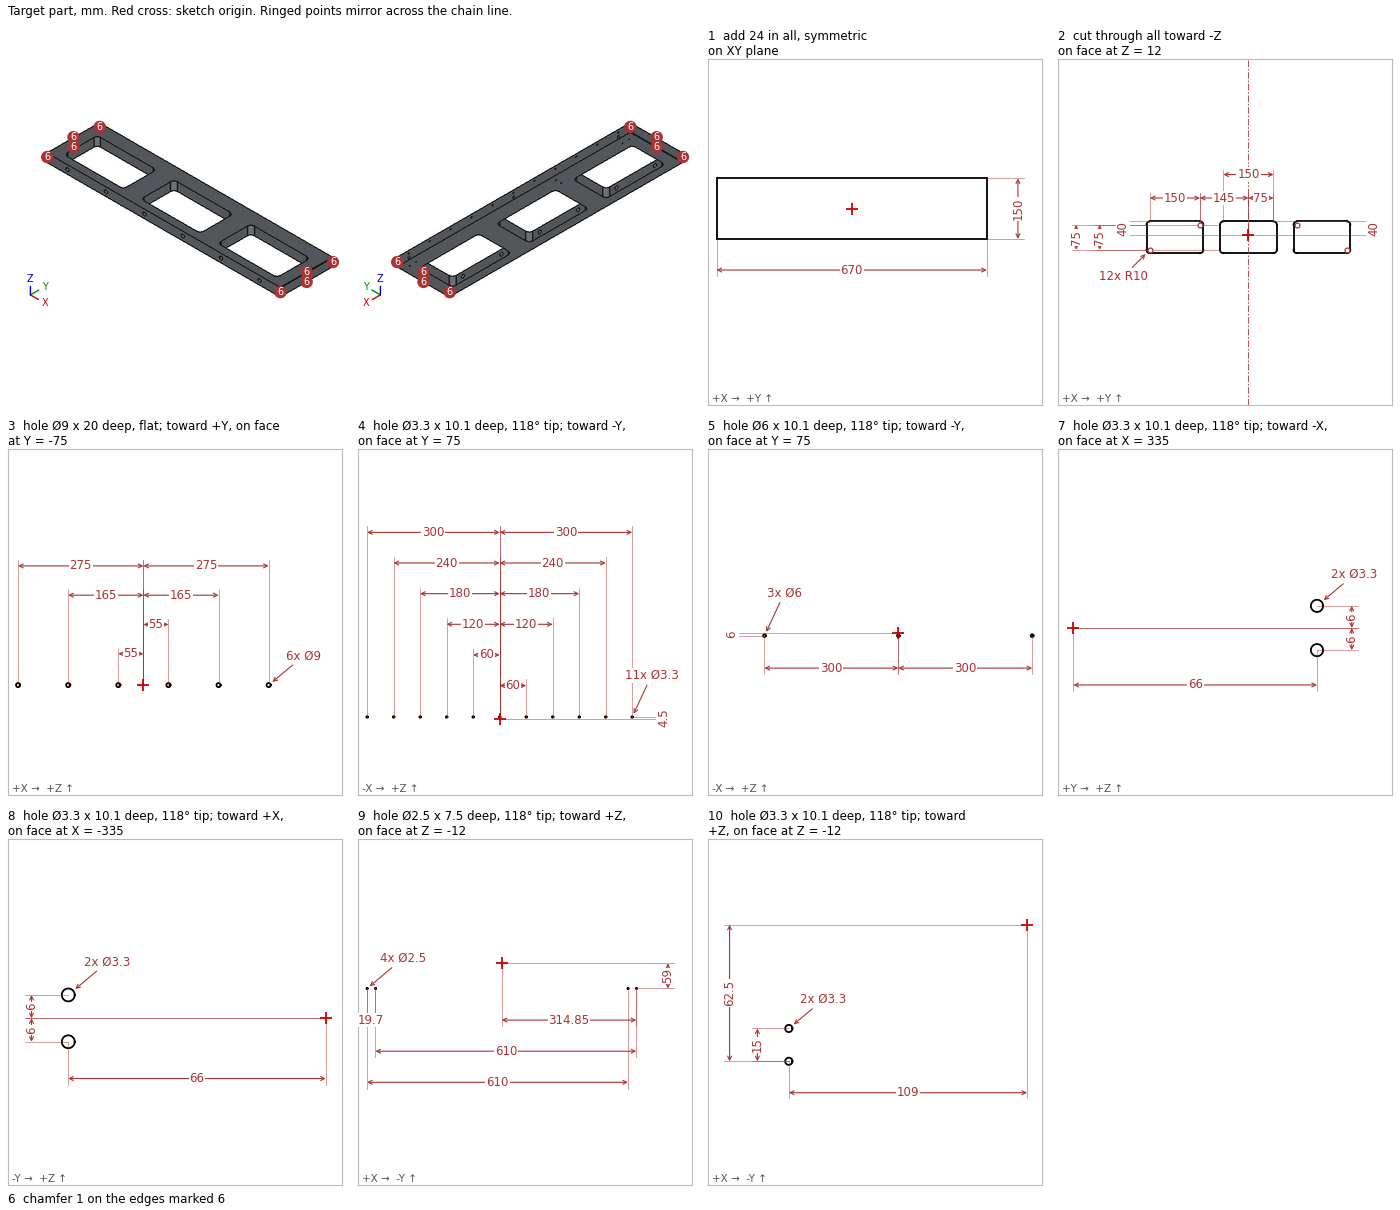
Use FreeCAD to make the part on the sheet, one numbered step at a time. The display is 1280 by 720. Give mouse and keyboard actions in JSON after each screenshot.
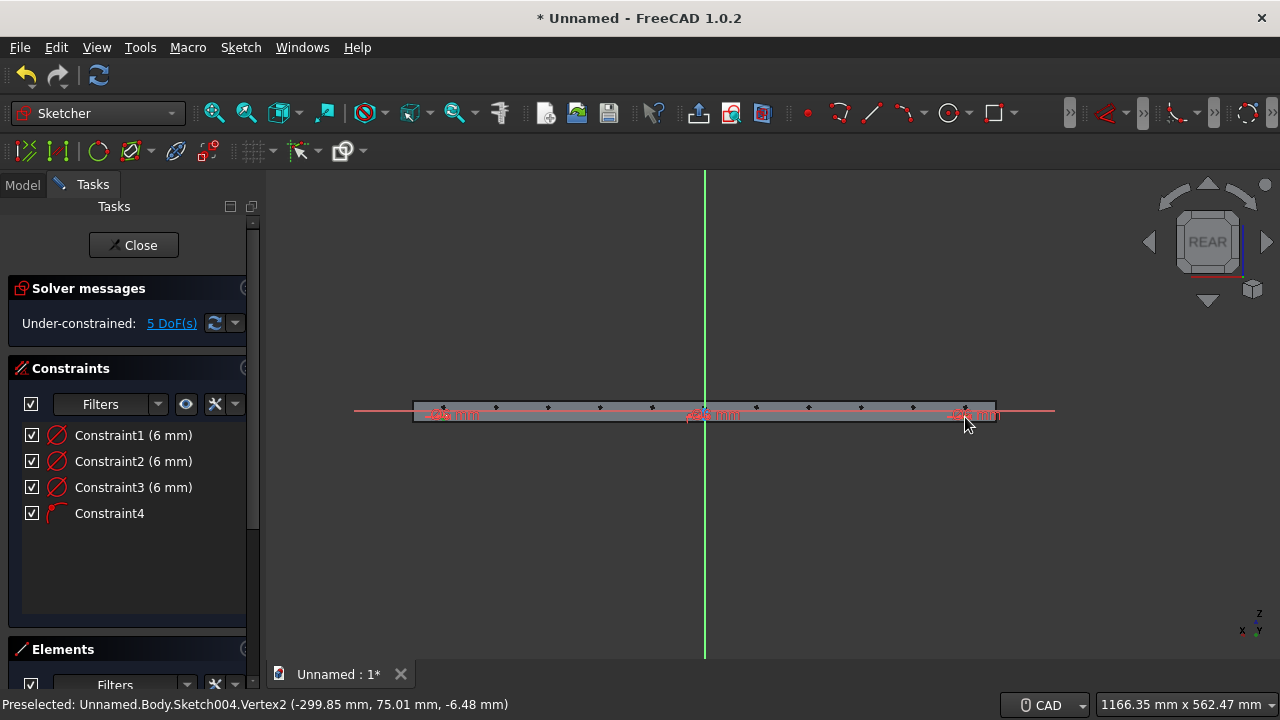
{"action": "key", "text": "h"}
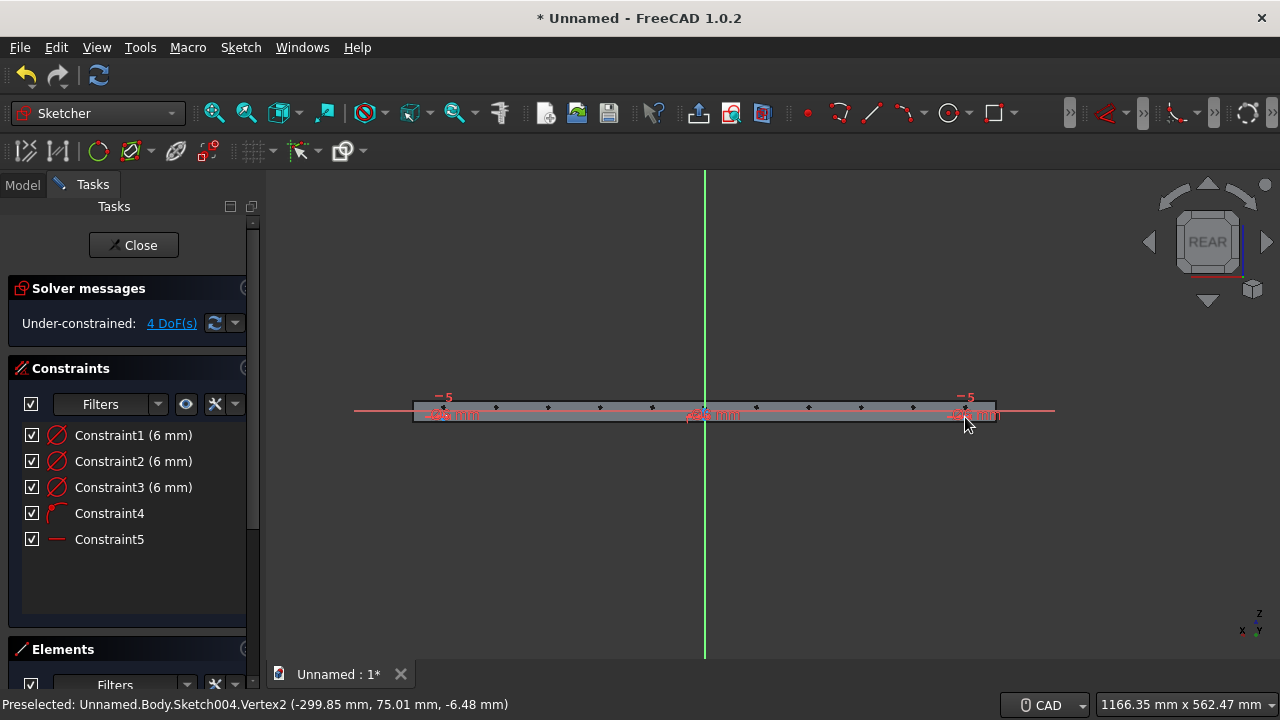
{"action": "left_click", "coordinate": [444, 417]}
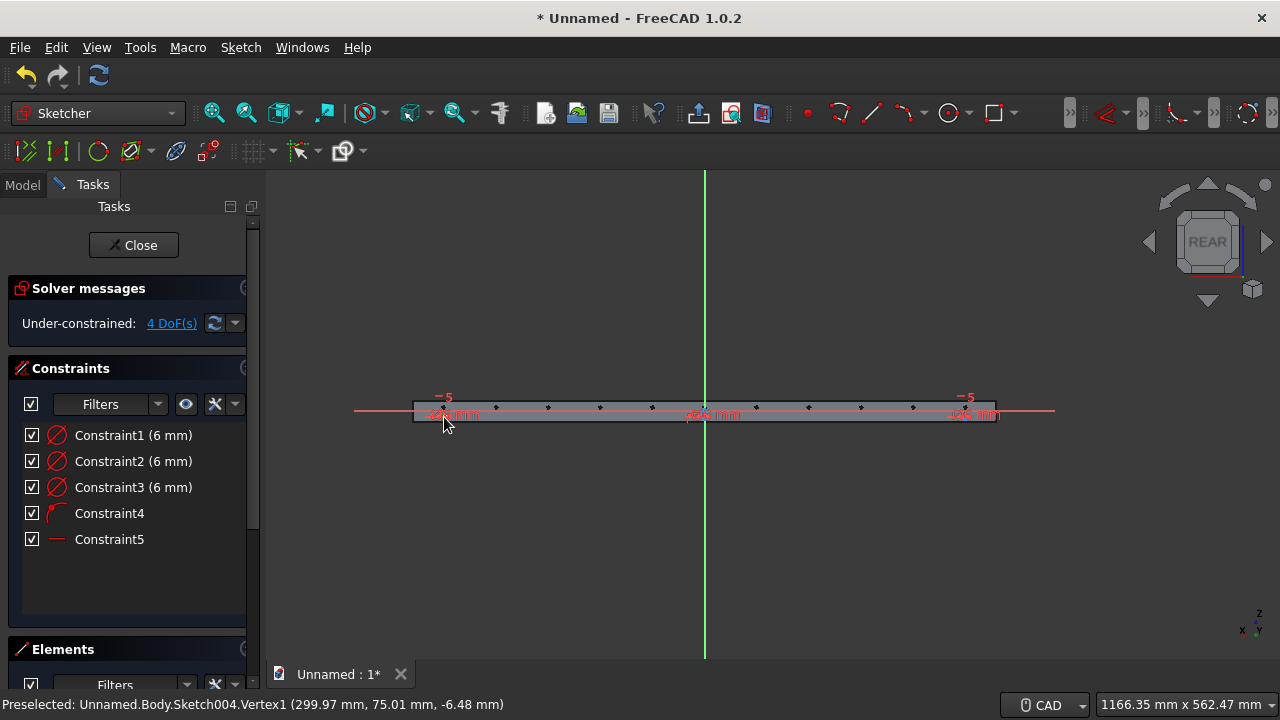
{"action": "scroll", "coordinate": [705, 417], "scroll_direction": "up", "scroll_amount": 4}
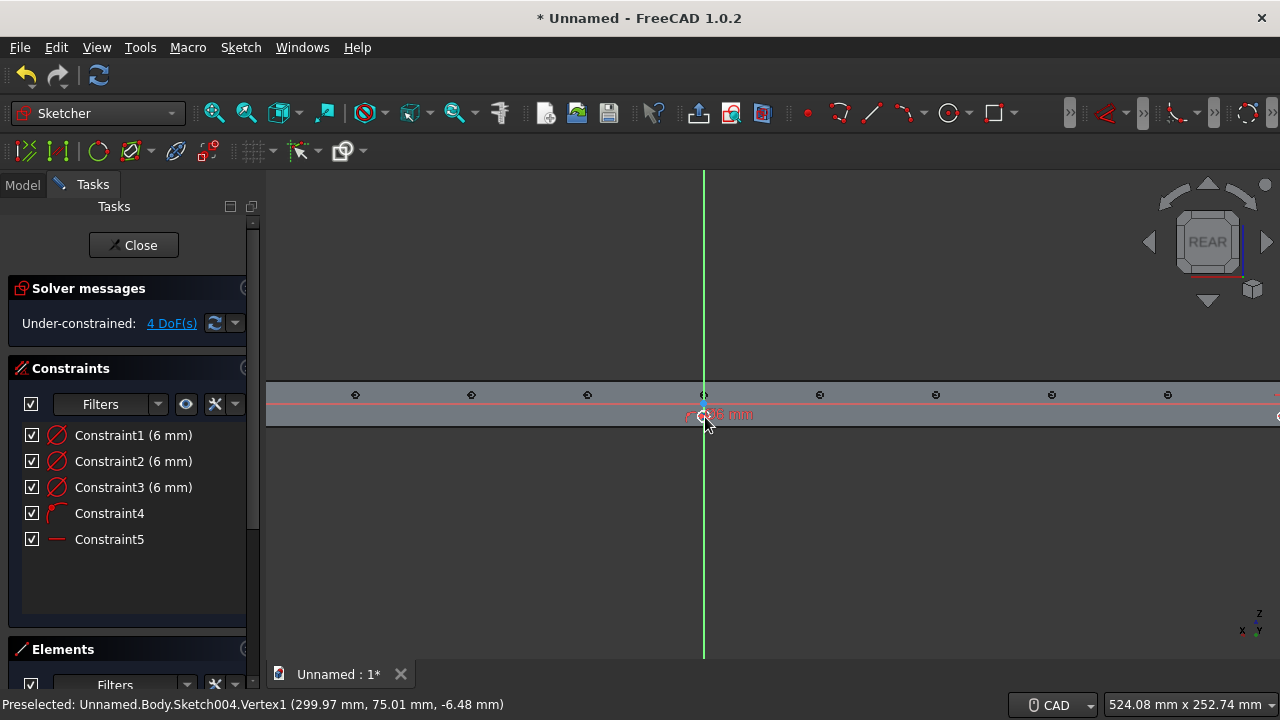
{"action": "left_click", "coordinate": [704, 416]}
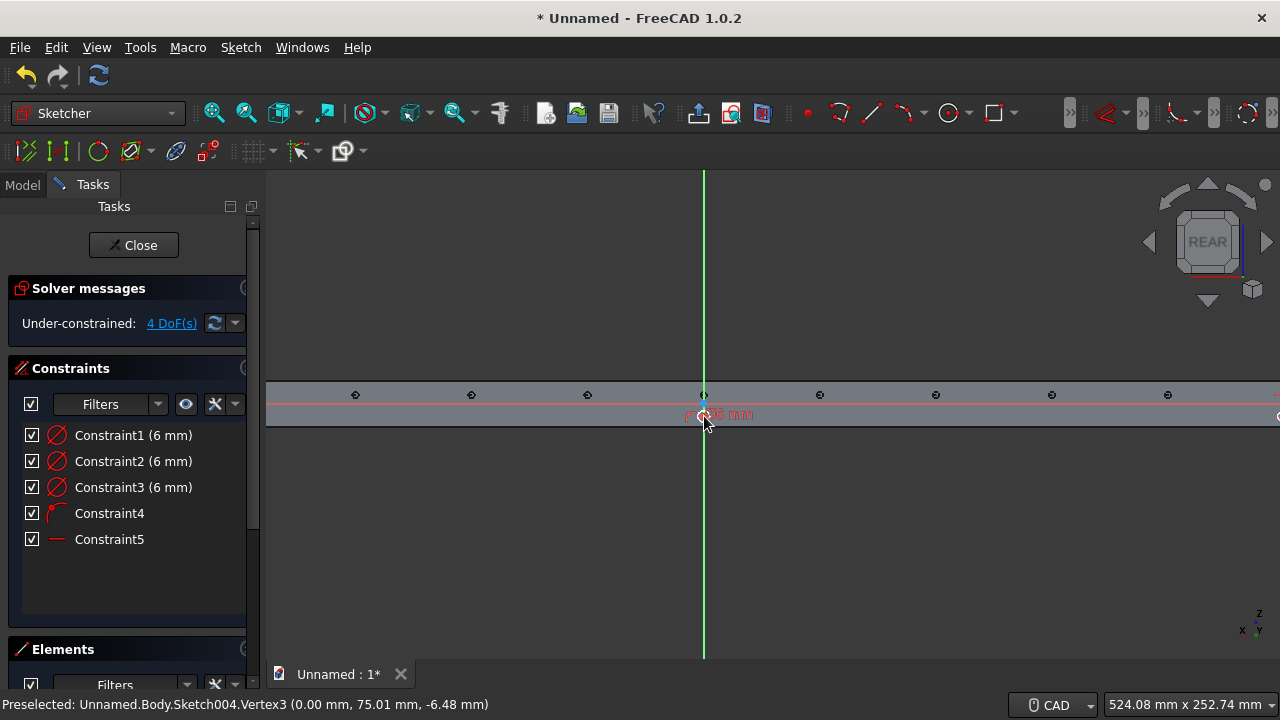
{"action": "key", "text": "h"}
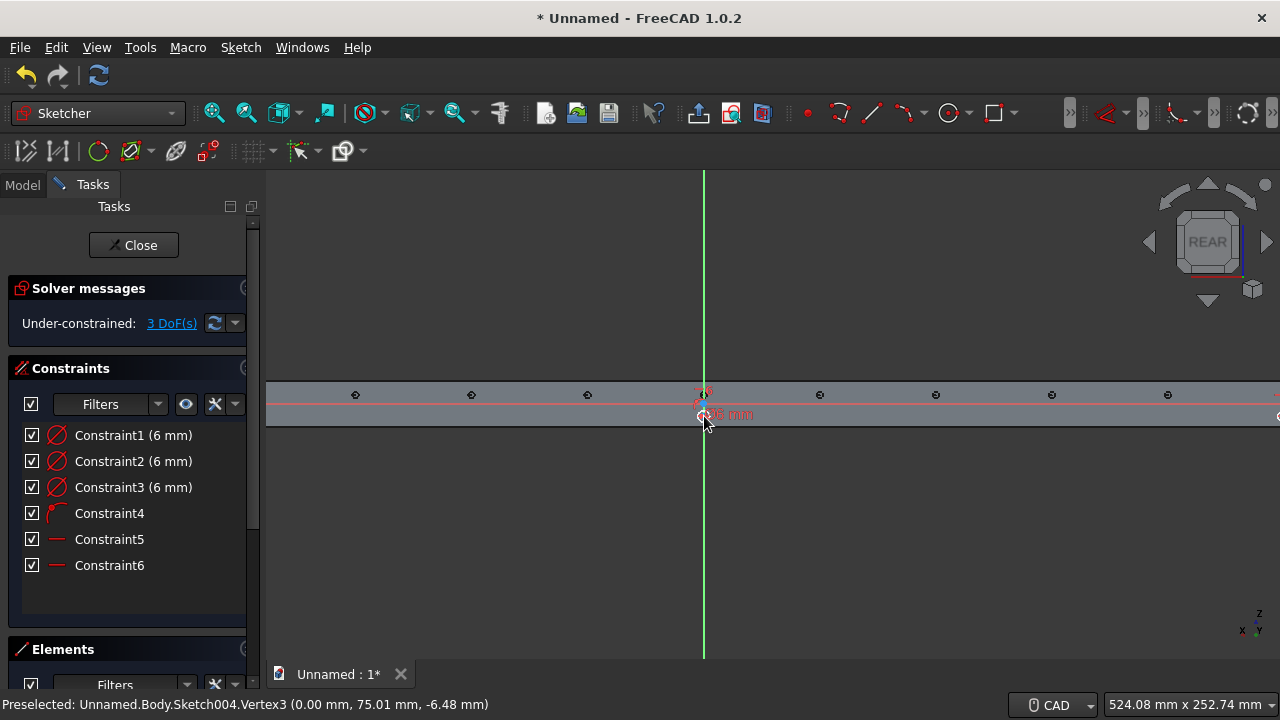
{"action": "left_click", "coordinate": [1106, 114]}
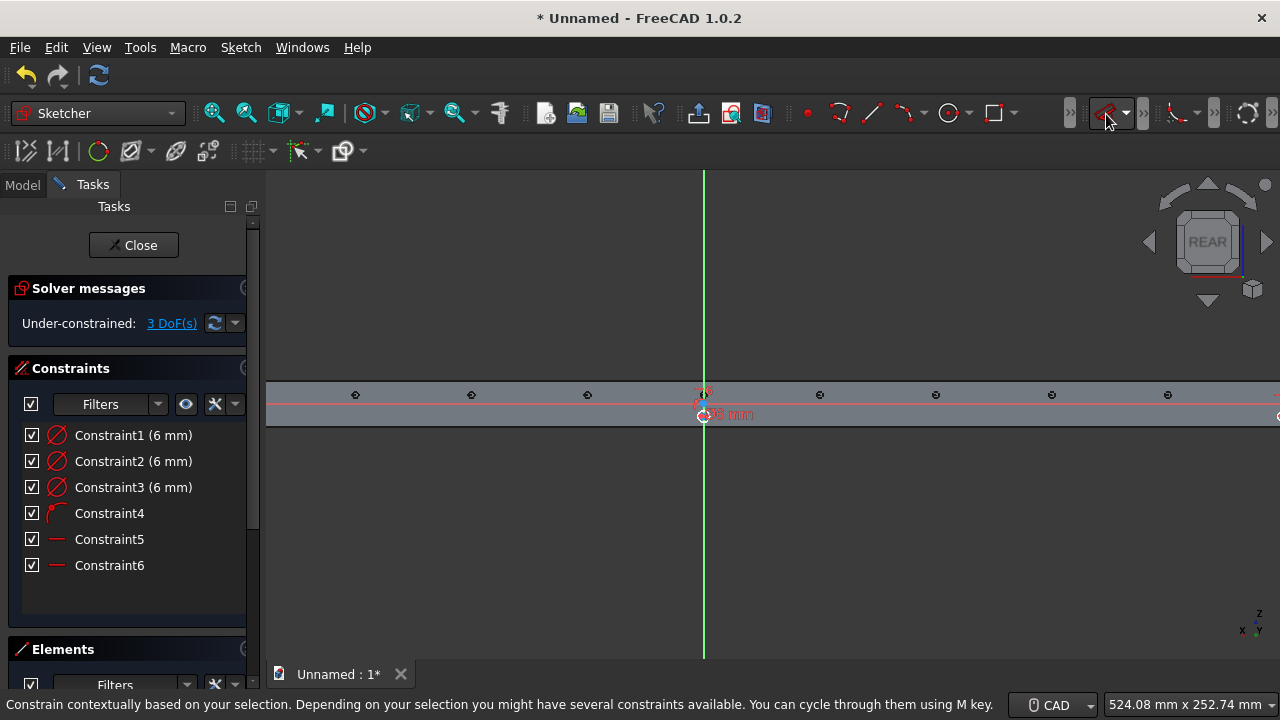
{"action": "scroll", "coordinate": [705, 416], "scroll_direction": "down", "scroll_amount": 4}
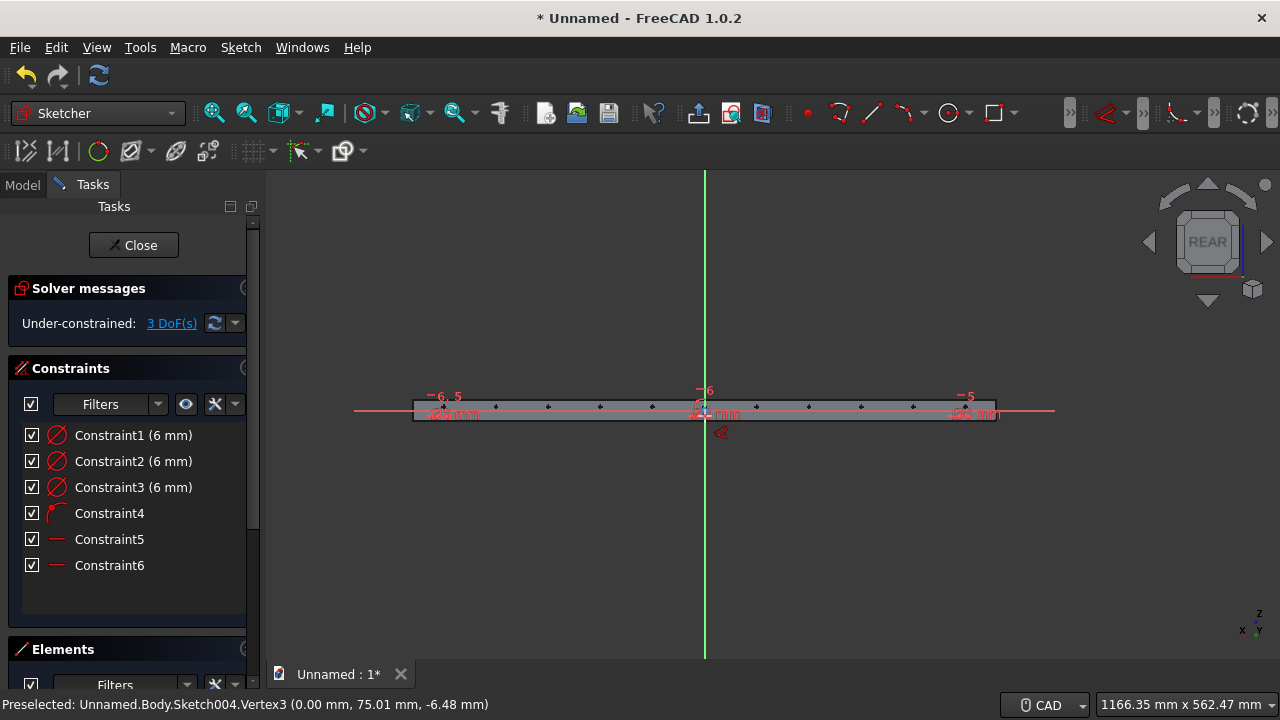
{"action": "scroll", "coordinate": [444, 416], "scroll_direction": "up", "scroll_amount": 11}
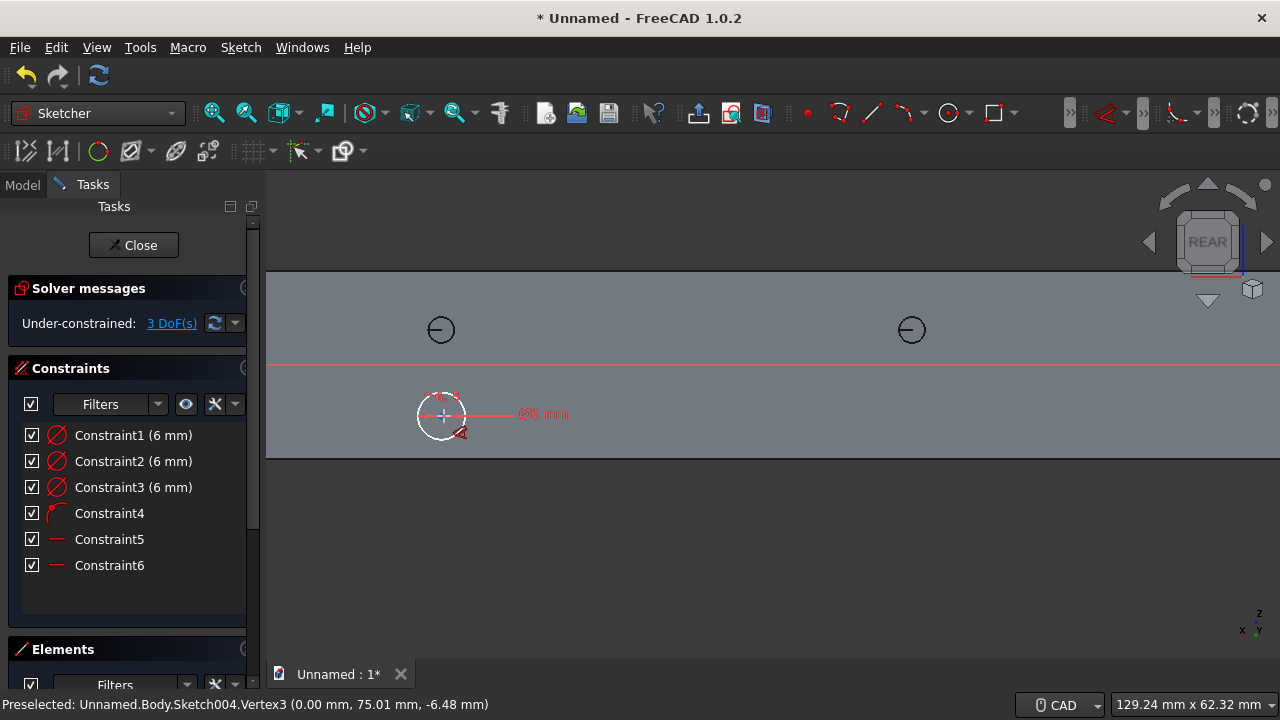
{"action": "left_click", "coordinate": [442, 416]}
{"action": "left_click", "coordinate": [408, 391]}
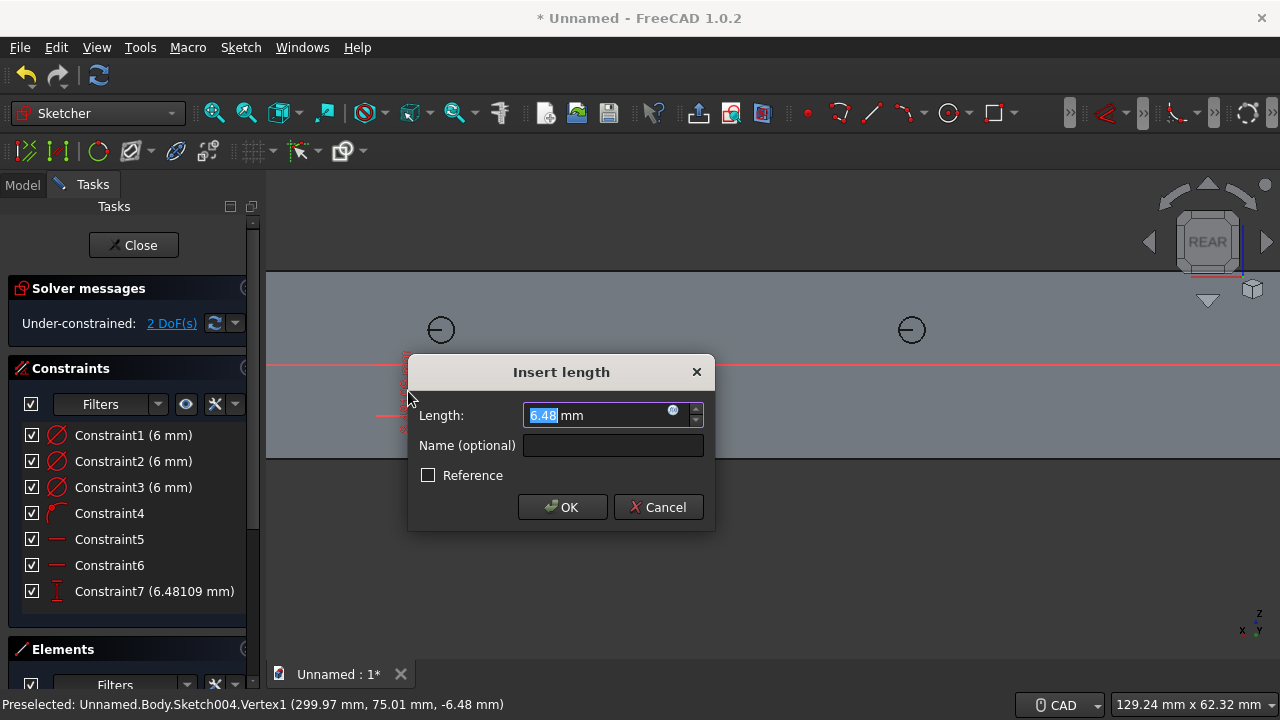
{"action": "type", "text": "6"}
{"action": "key", "text": "Return"}